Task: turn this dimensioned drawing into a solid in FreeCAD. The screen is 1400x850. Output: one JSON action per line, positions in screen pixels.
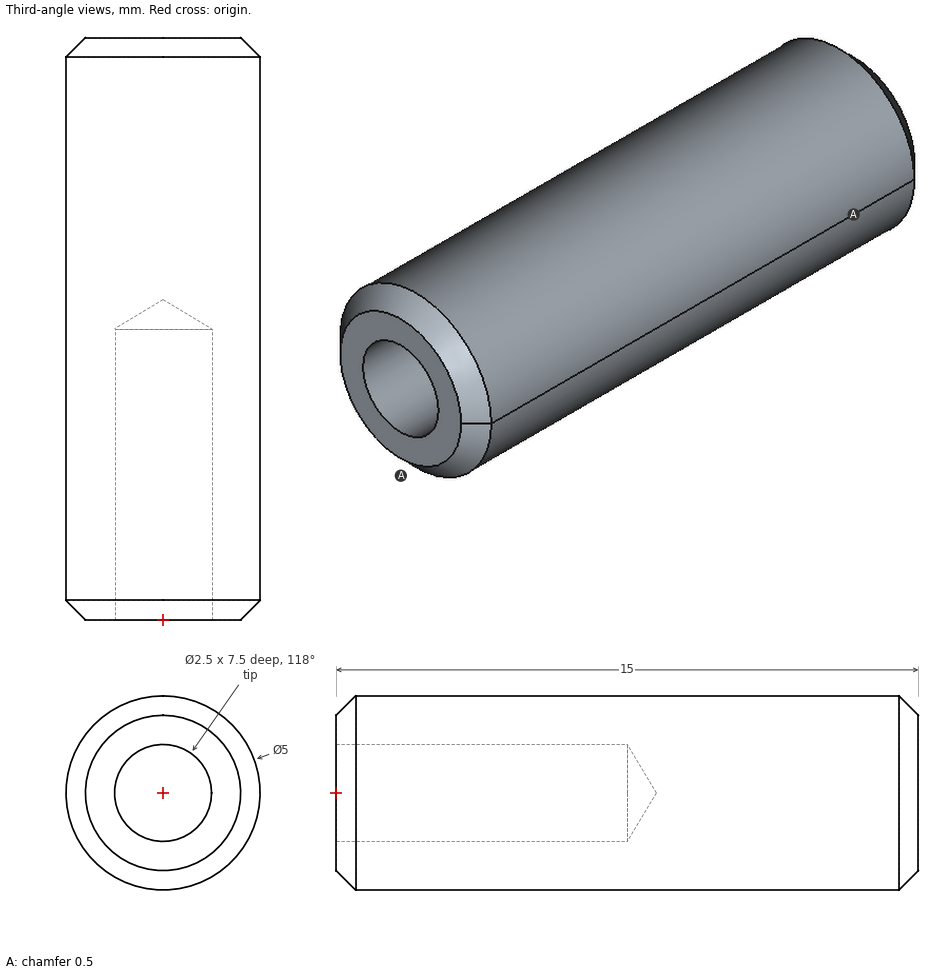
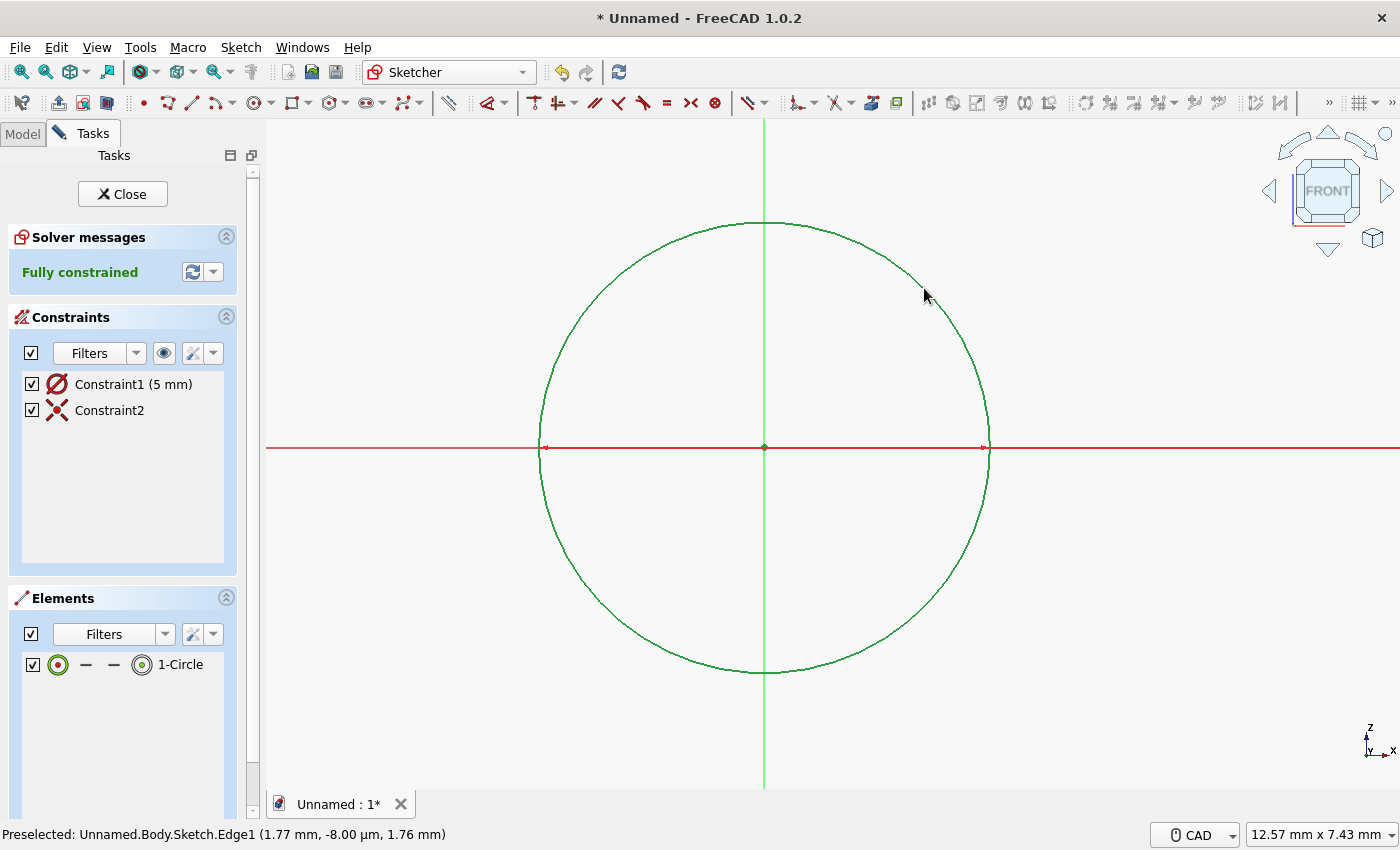
{"action": "left_click", "coordinate": [123, 194]}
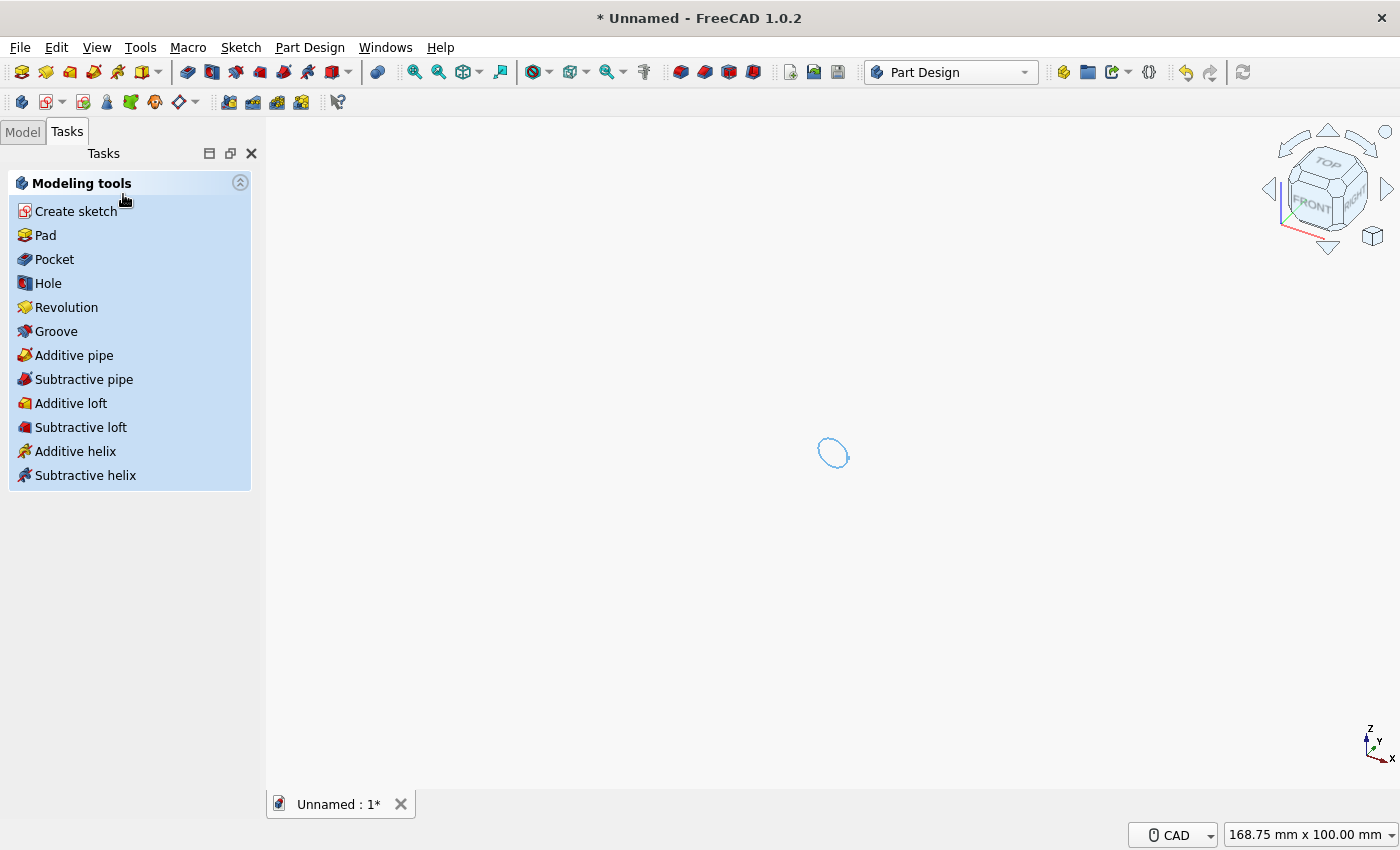
{"action": "left_click", "coordinate": [22, 72]}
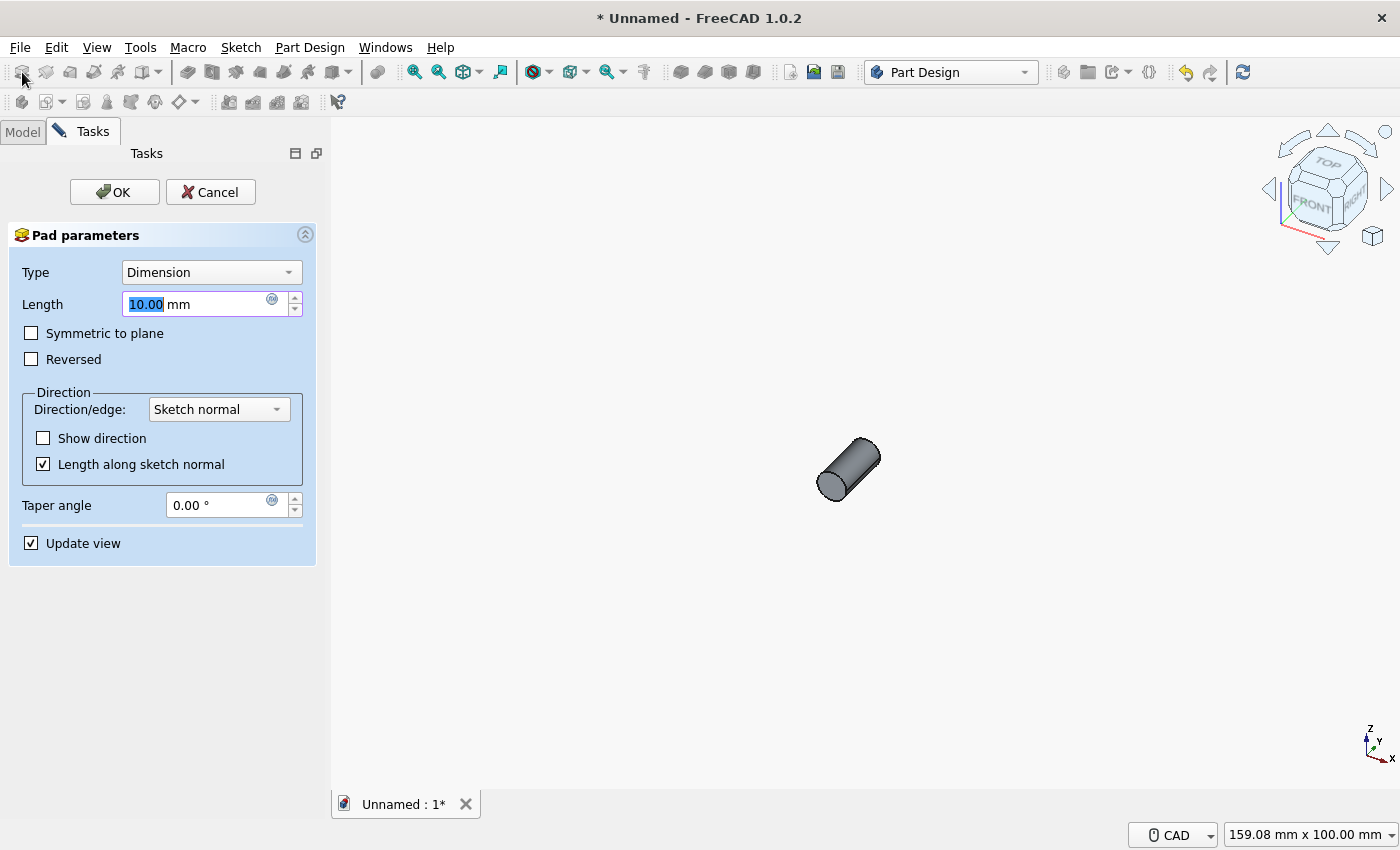
{"action": "type", "text": "15"}
{"action": "key", "text": "Tab"}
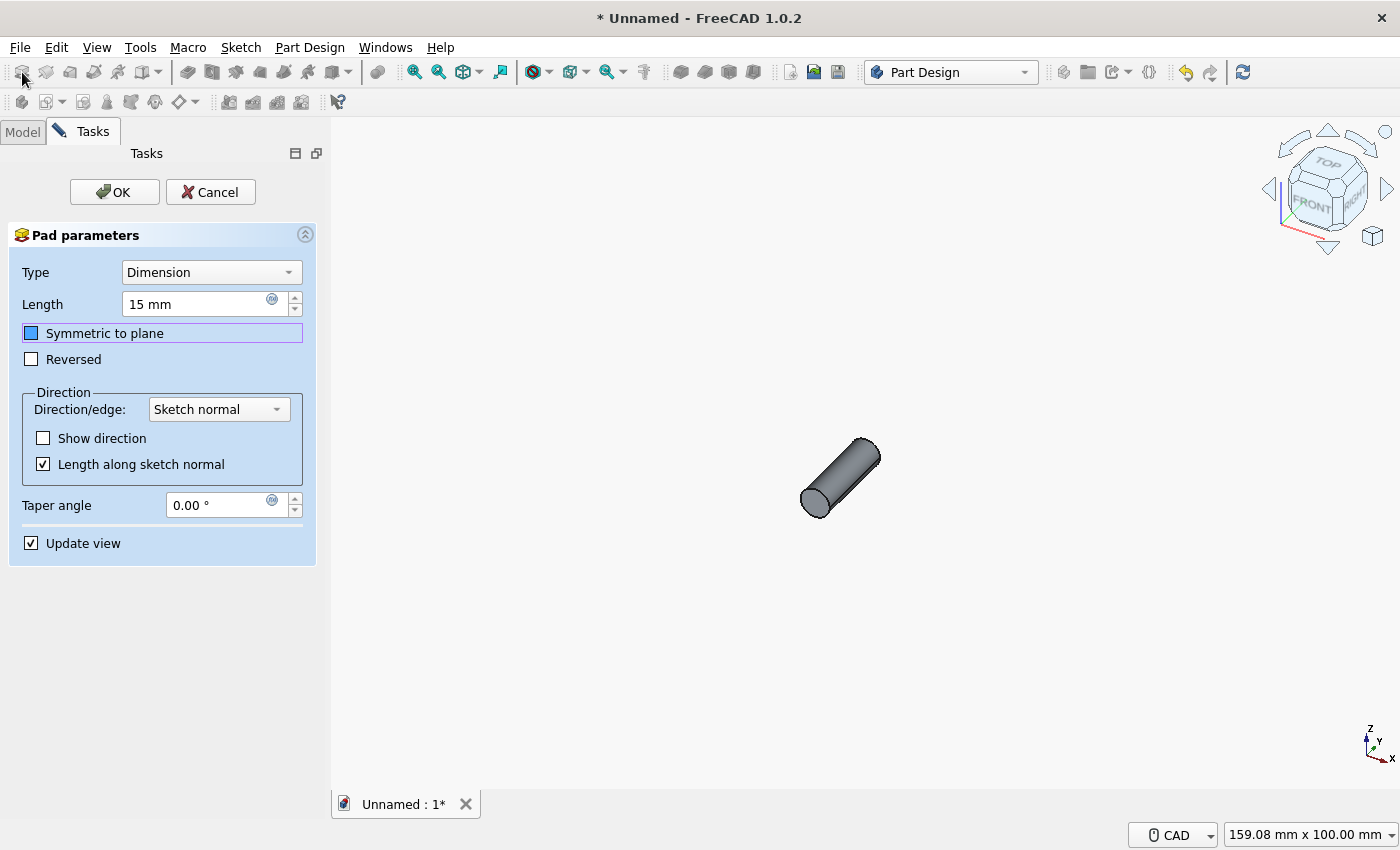
{"action": "left_click", "coordinate": [30, 359]}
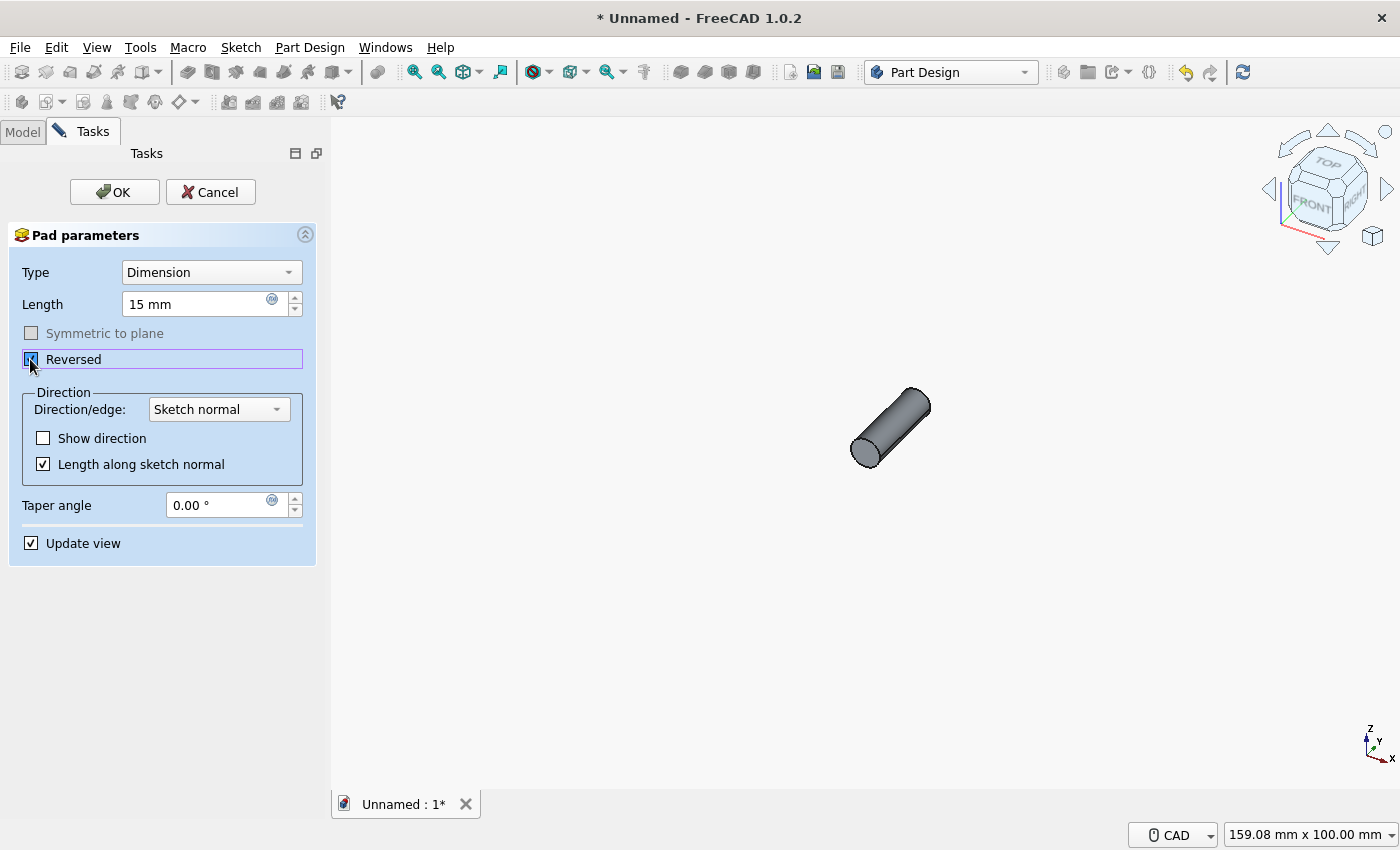
{"action": "left_click", "coordinate": [115, 192]}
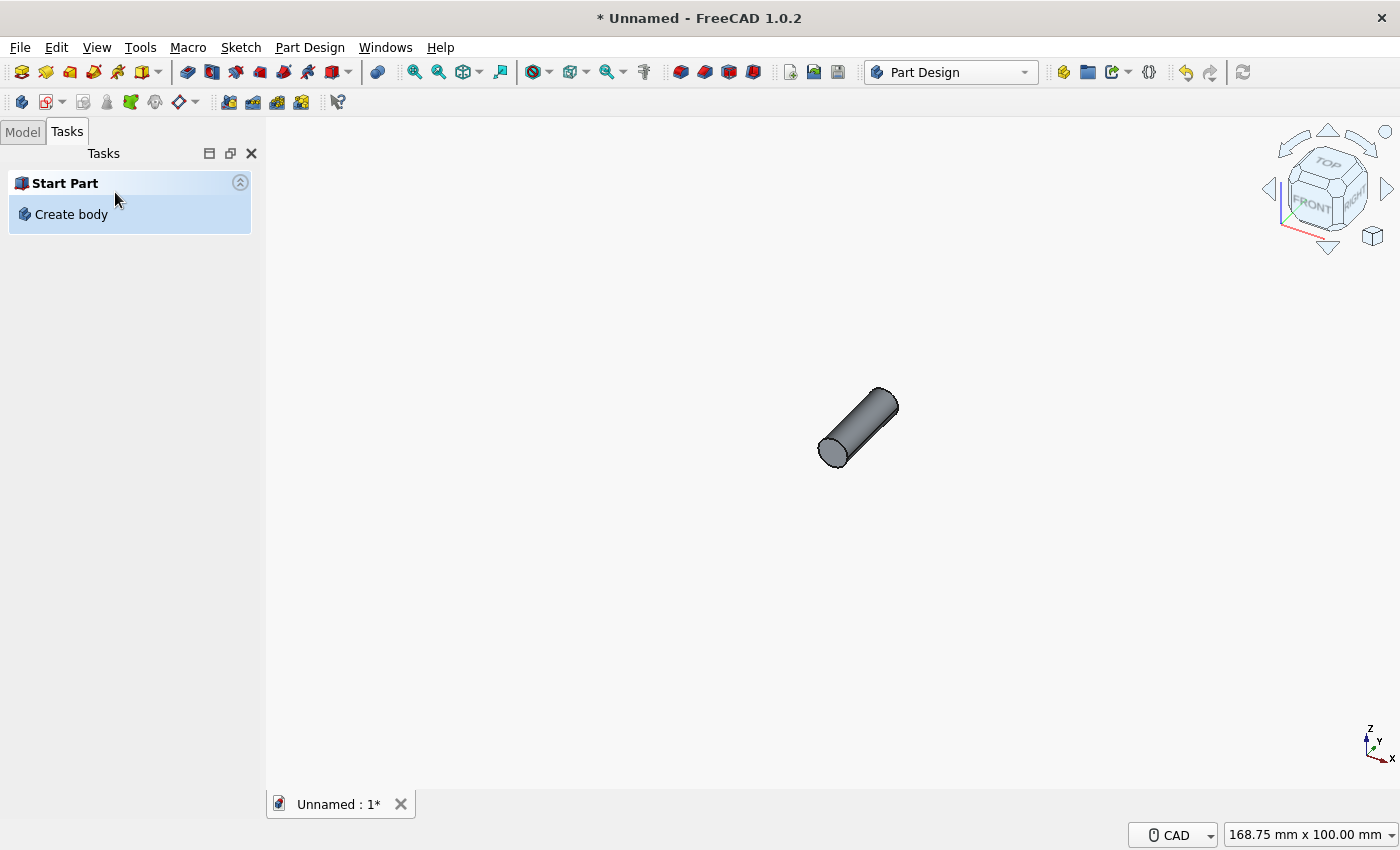
{"action": "left_click", "coordinate": [416, 72]}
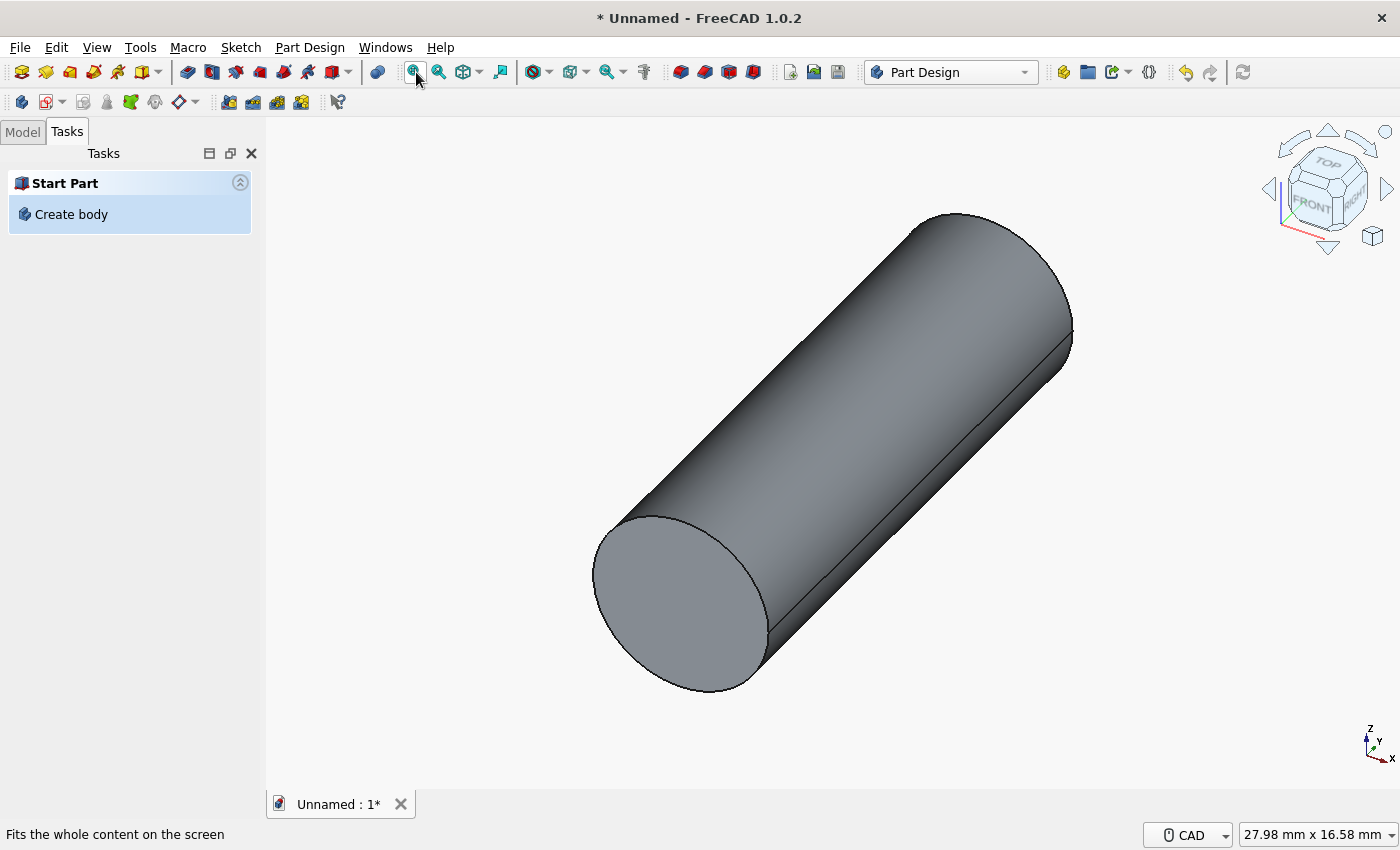
{"action": "left_click", "coordinate": [681, 603]}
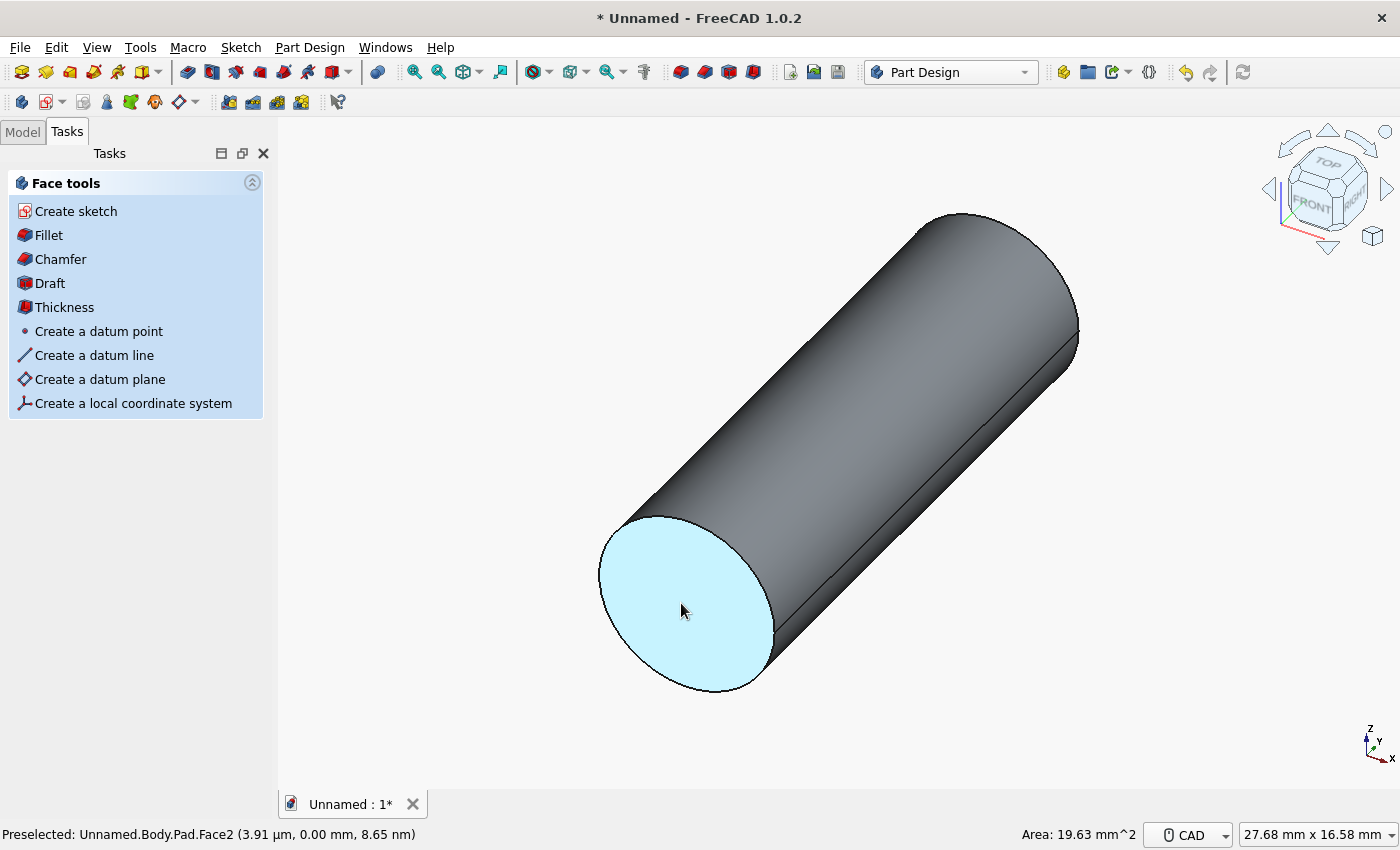
{"action": "left_click", "coordinate": [46, 102]}